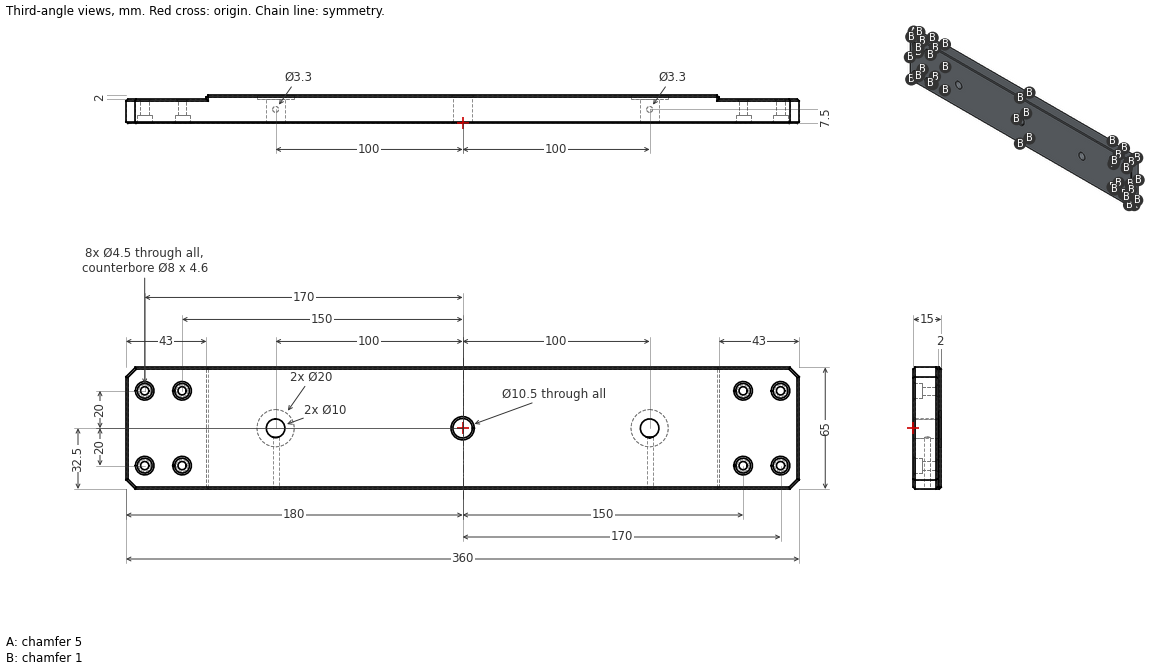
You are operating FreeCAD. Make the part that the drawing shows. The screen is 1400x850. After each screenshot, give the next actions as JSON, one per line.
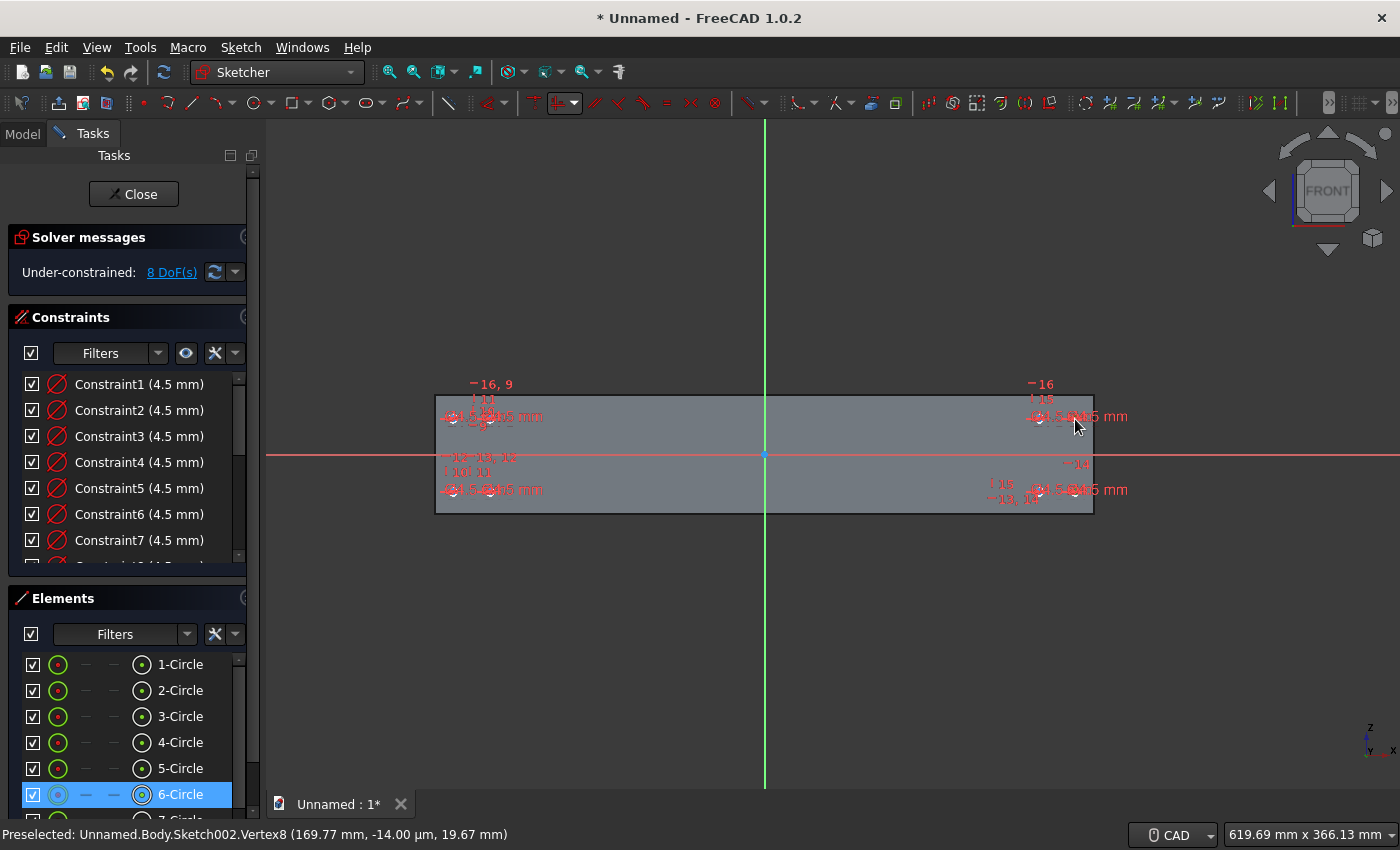
{"action": "key", "text": "v"}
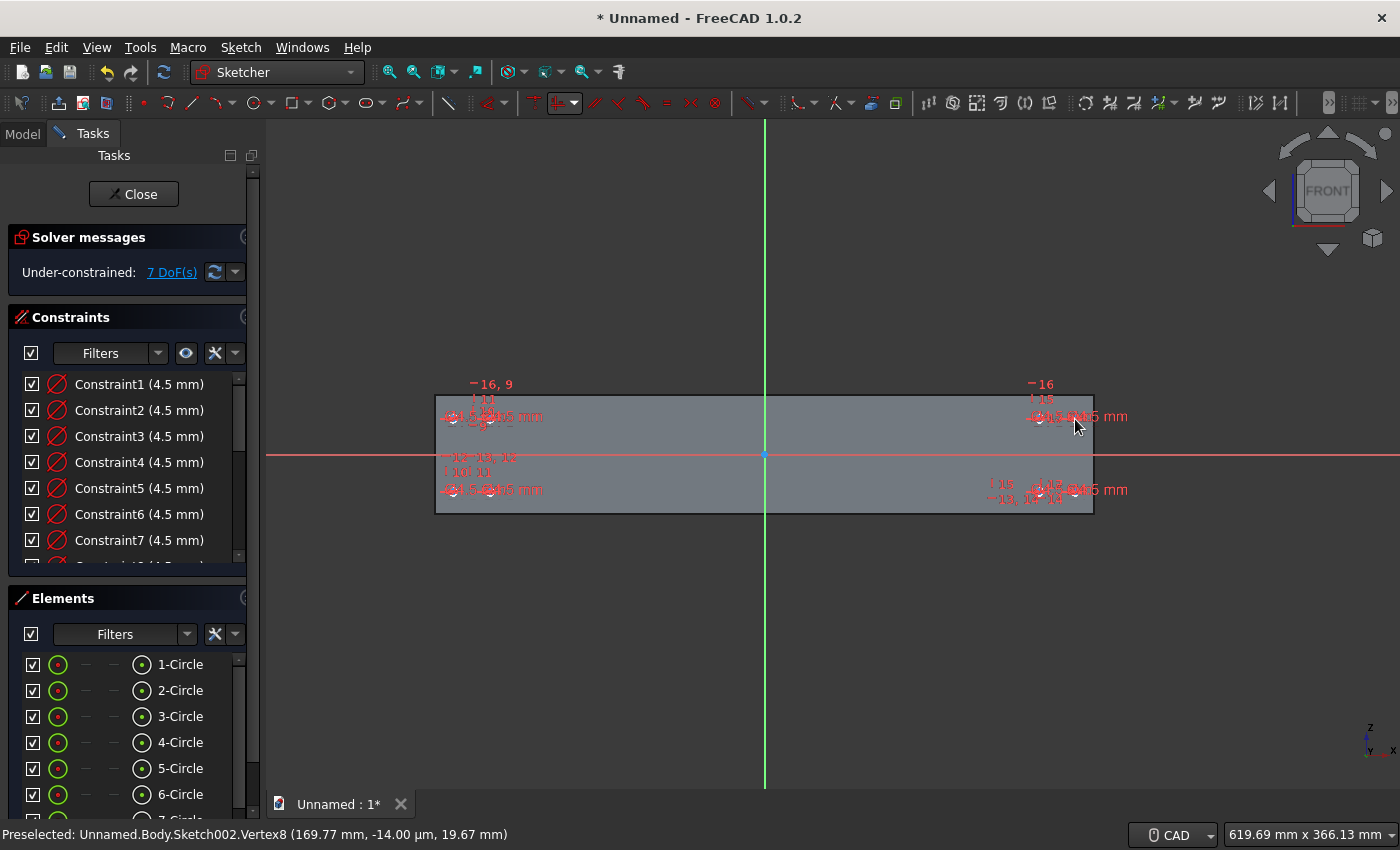
{"action": "scroll", "coordinate": [1039, 419], "scroll_direction": "up", "scroll_amount": 4}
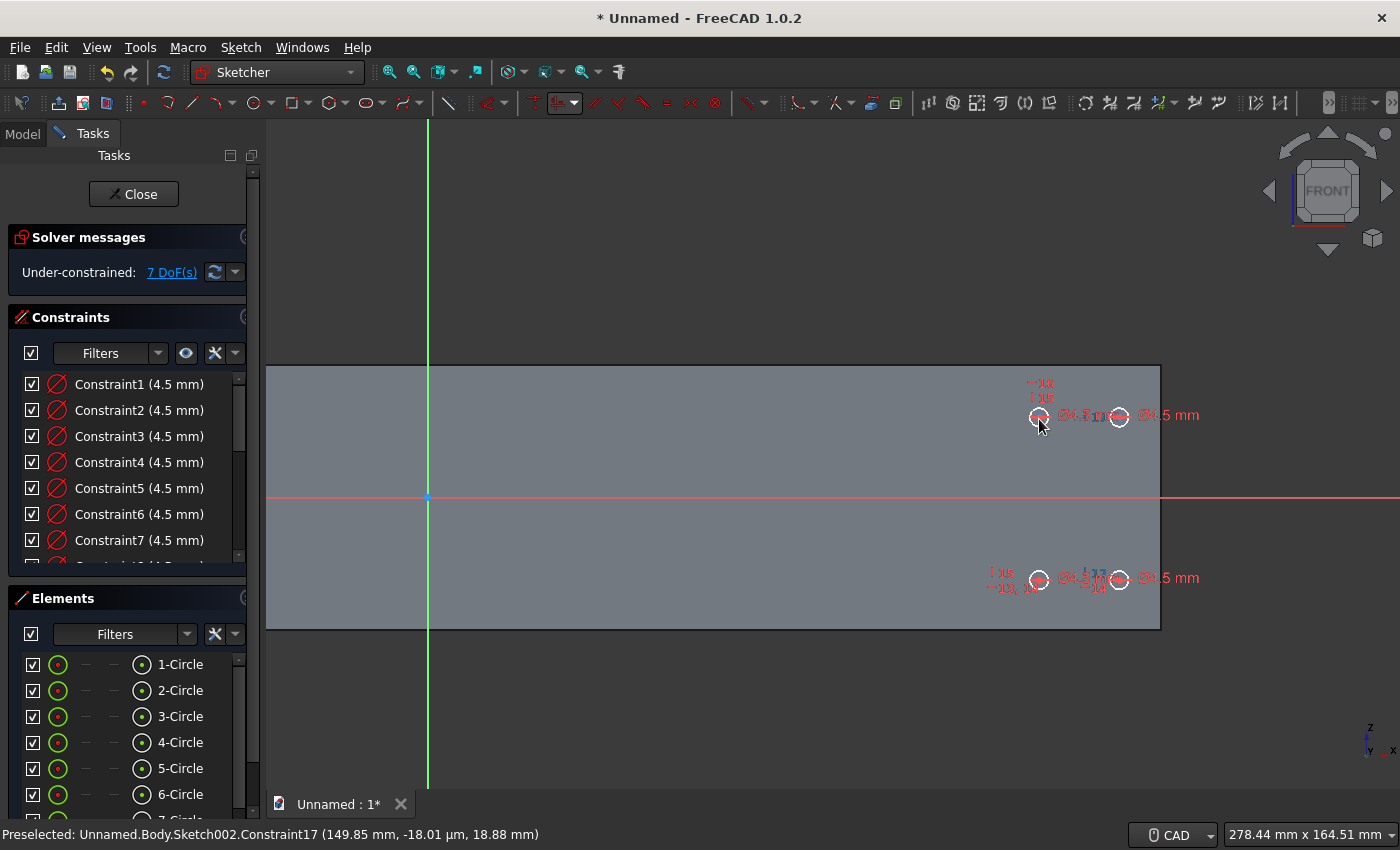
{"action": "left_click", "coordinate": [1039, 417]}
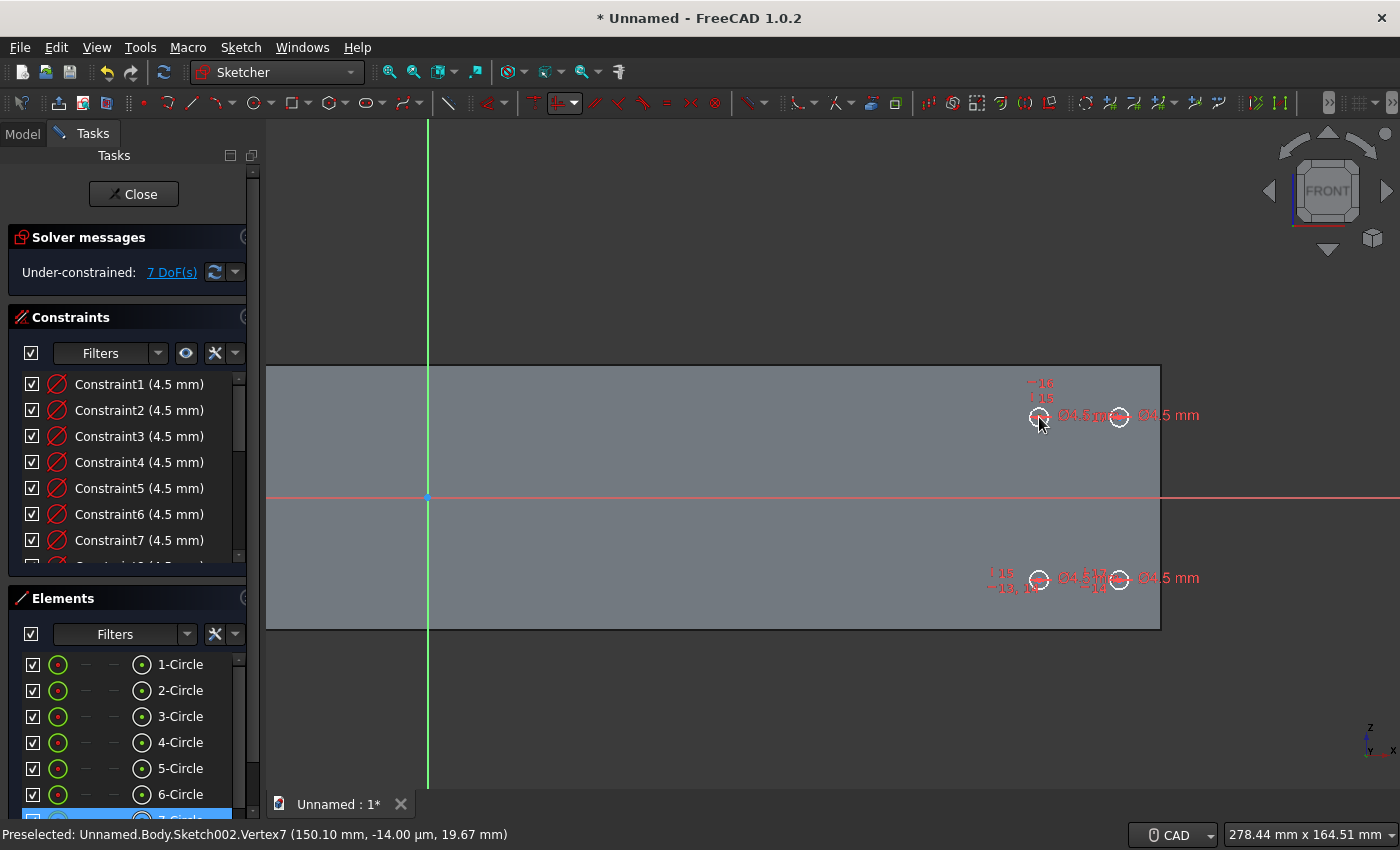
{"action": "left_click", "coordinate": [1119, 417]}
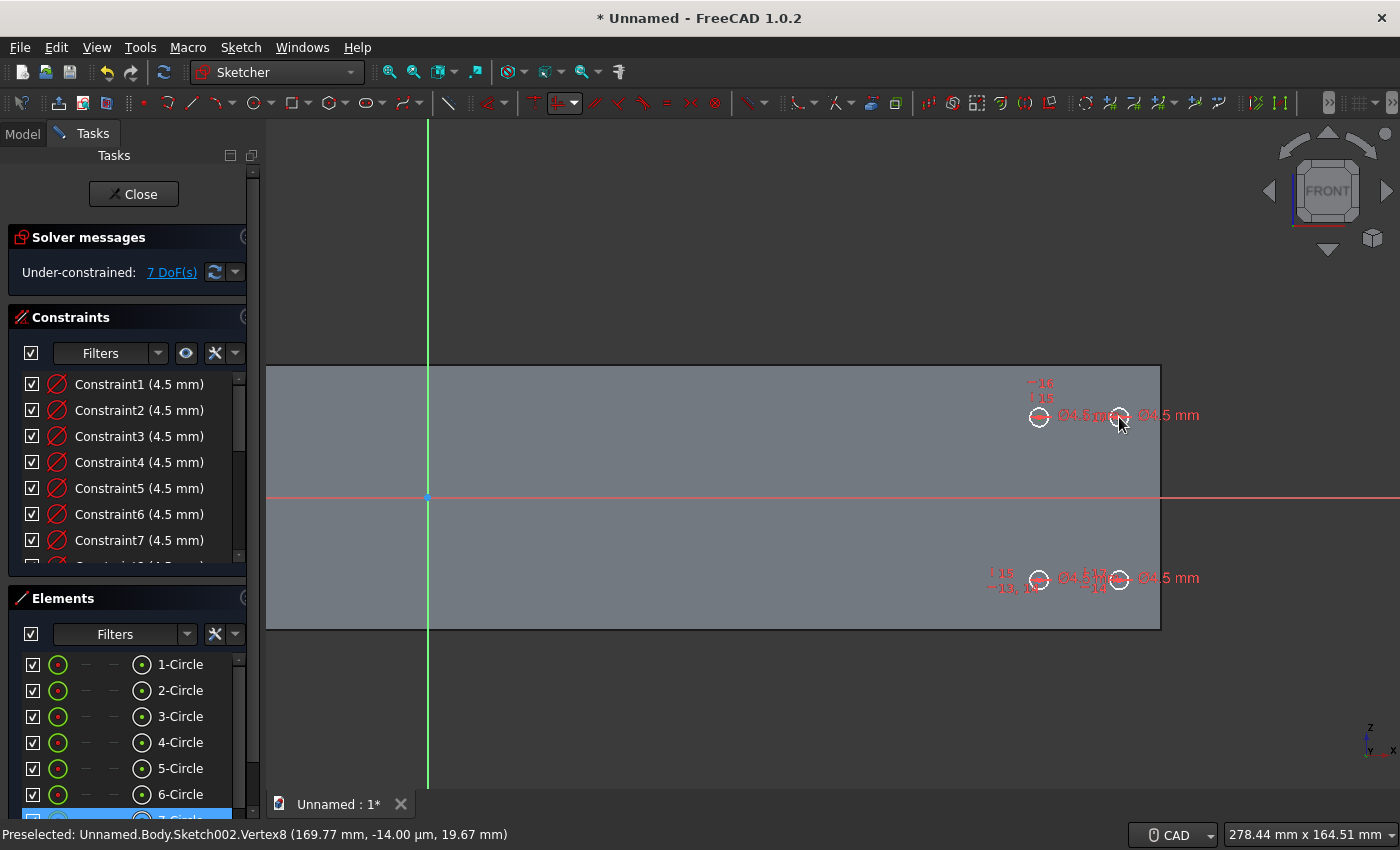
{"action": "key", "text": "h"}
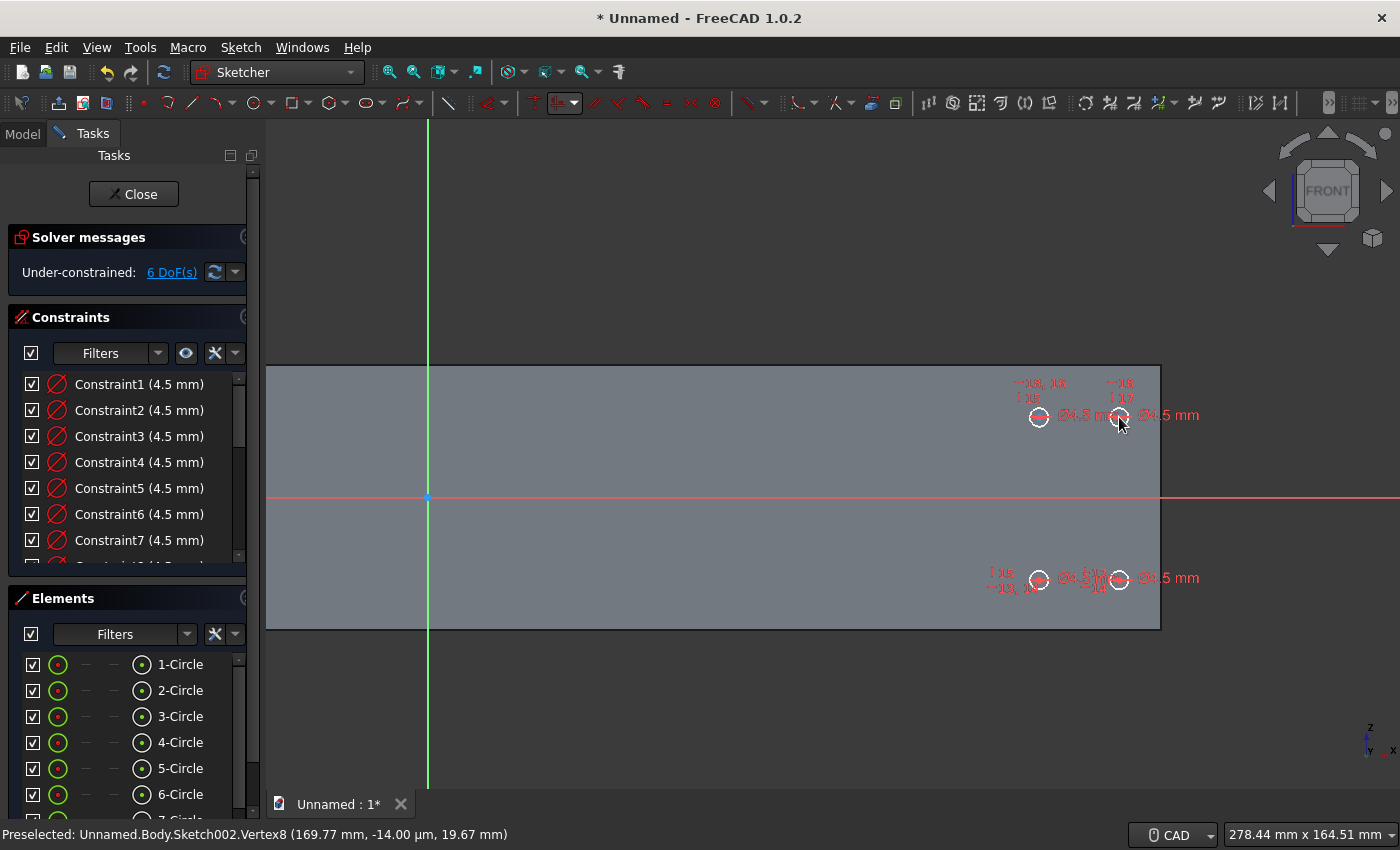
{"action": "left_click", "coordinate": [488, 104]}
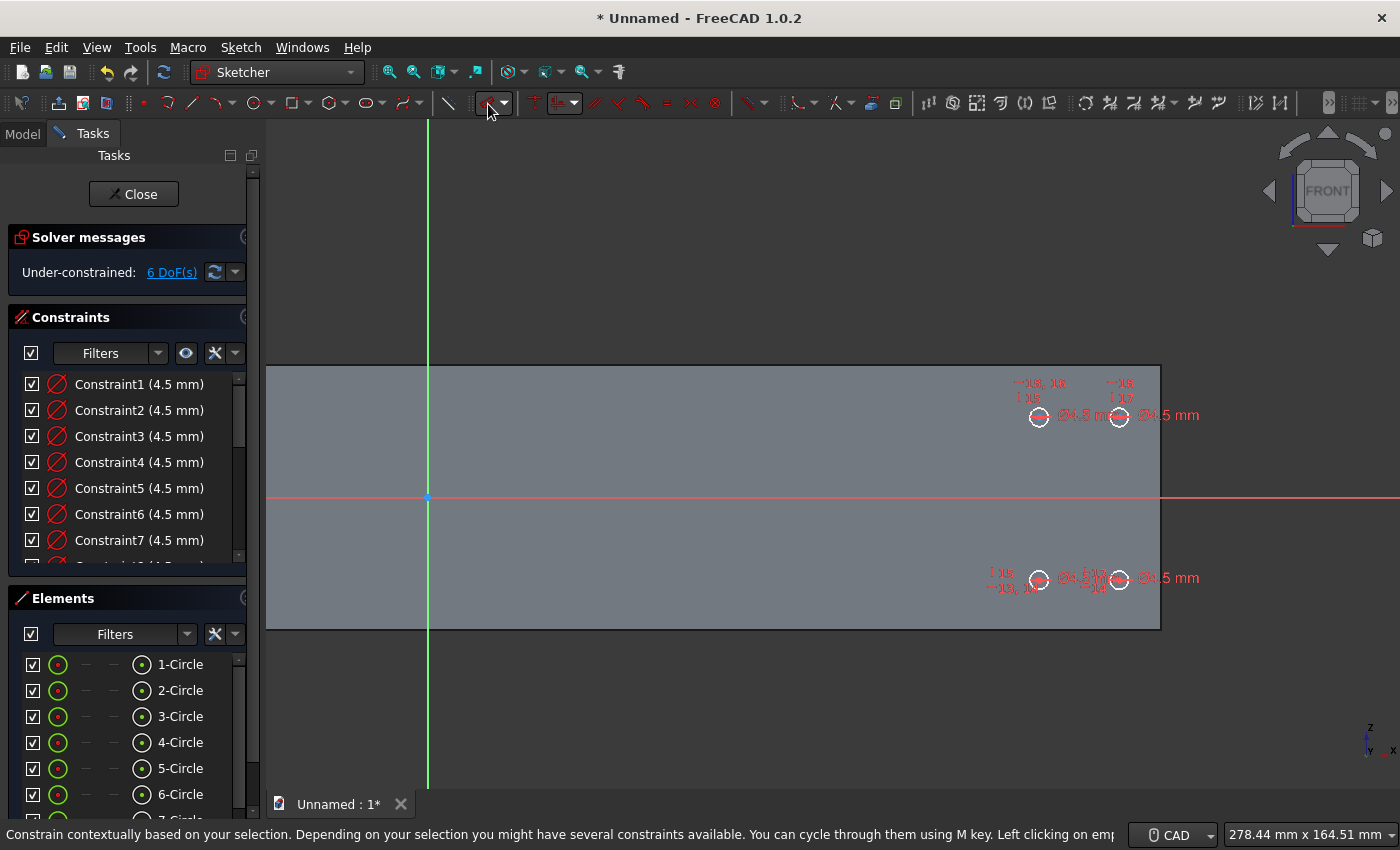
{"action": "scroll", "coordinate": [1039, 418], "scroll_direction": "down", "scroll_amount": 4}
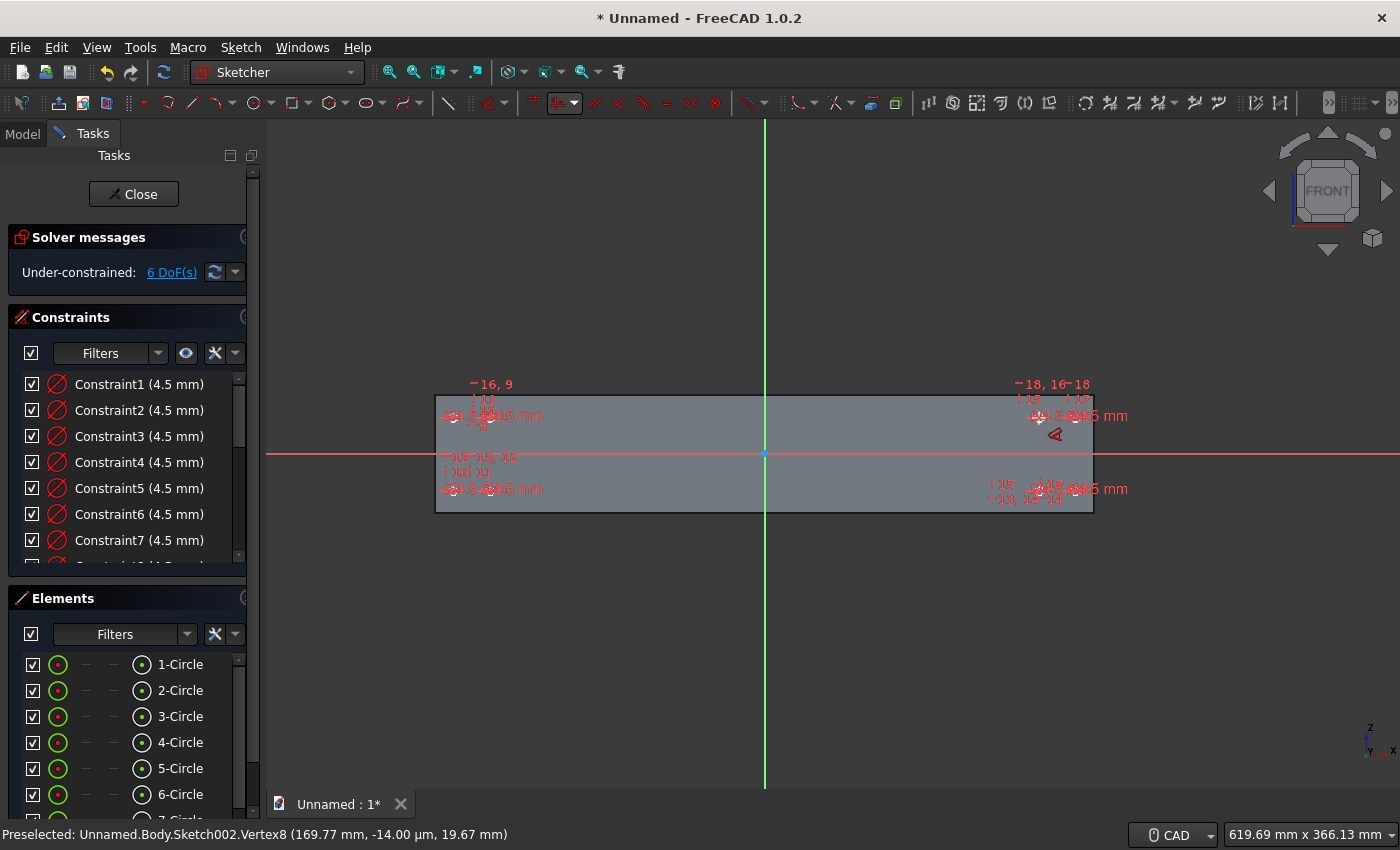
{"action": "left_click", "coordinate": [453, 418]}
{"action": "left_click", "coordinate": [419, 436]}